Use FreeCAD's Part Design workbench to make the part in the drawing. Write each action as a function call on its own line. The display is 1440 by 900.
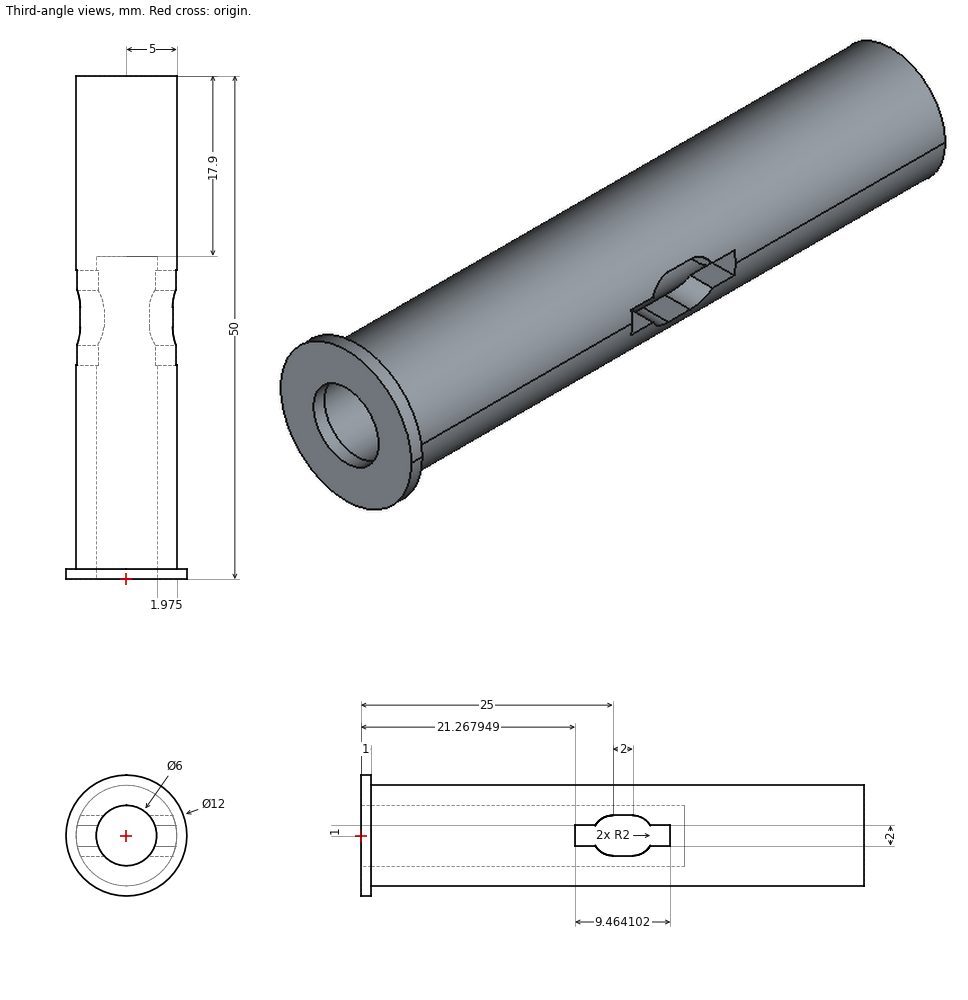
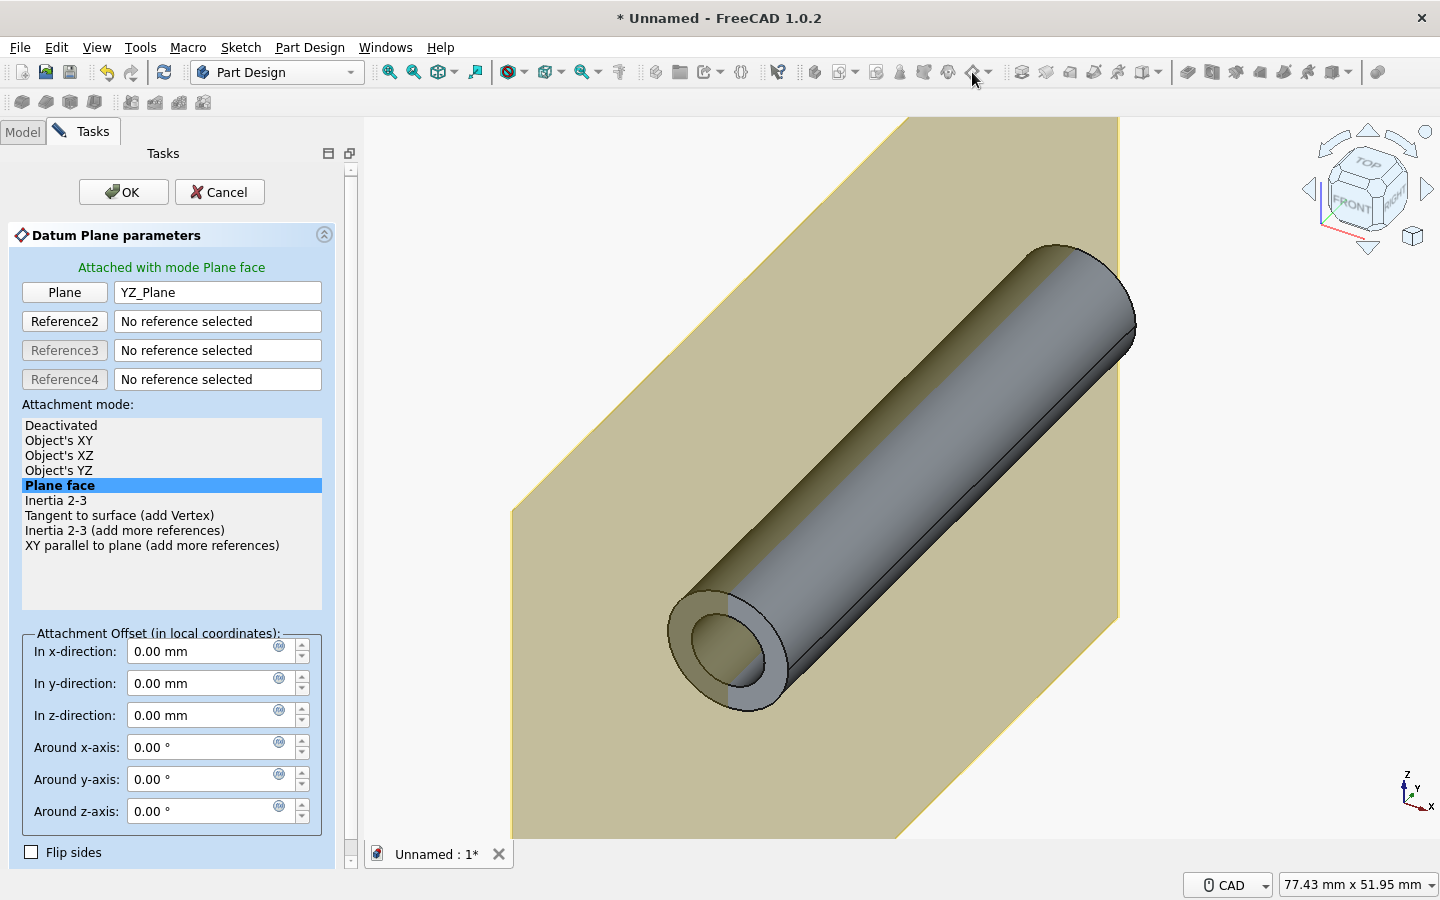
triple_click(210, 715)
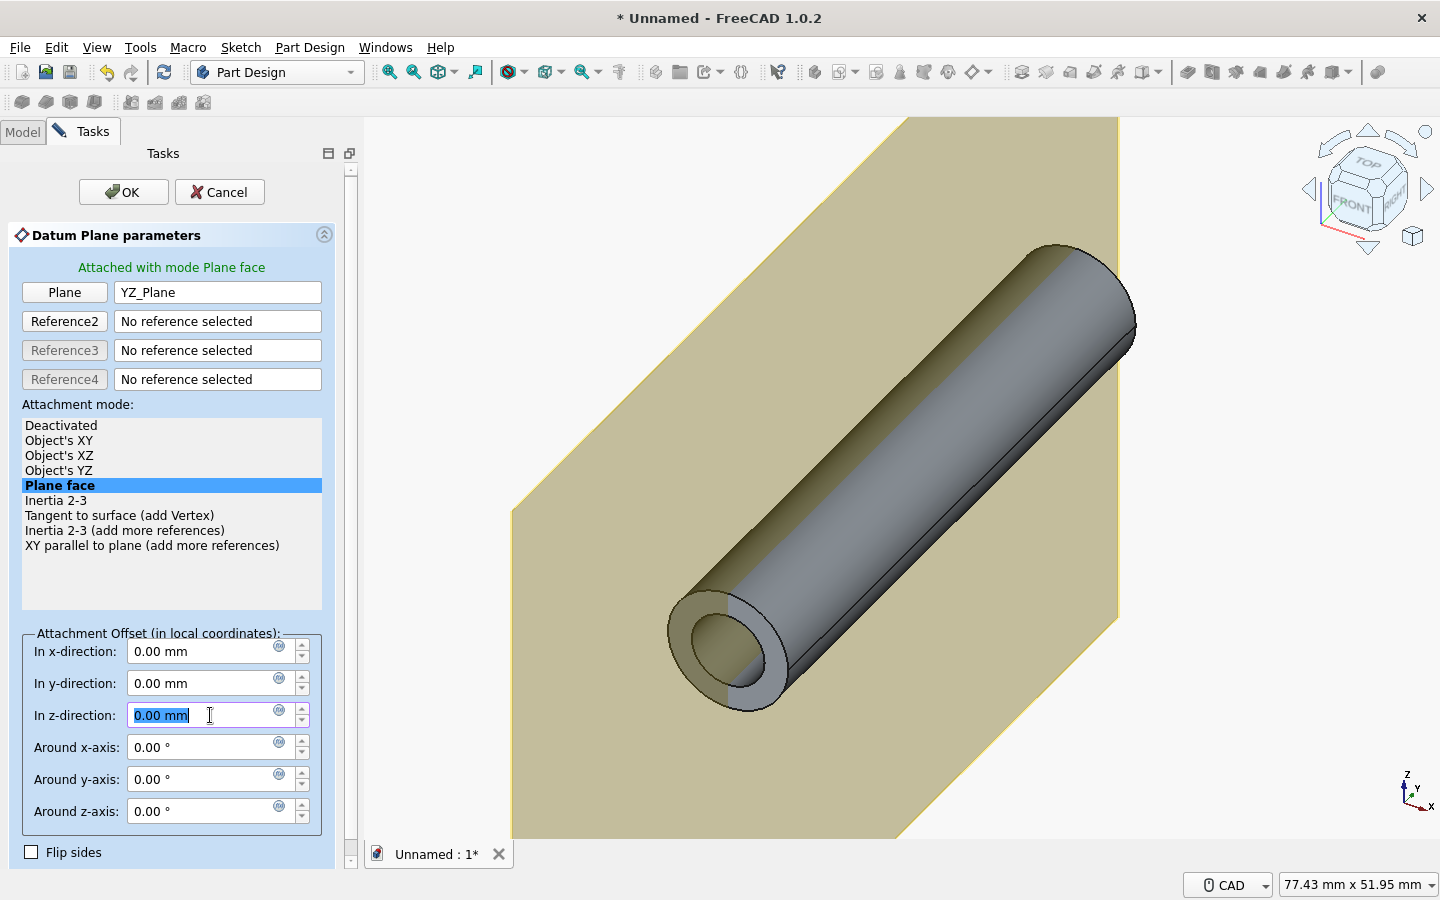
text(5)
key(Tab)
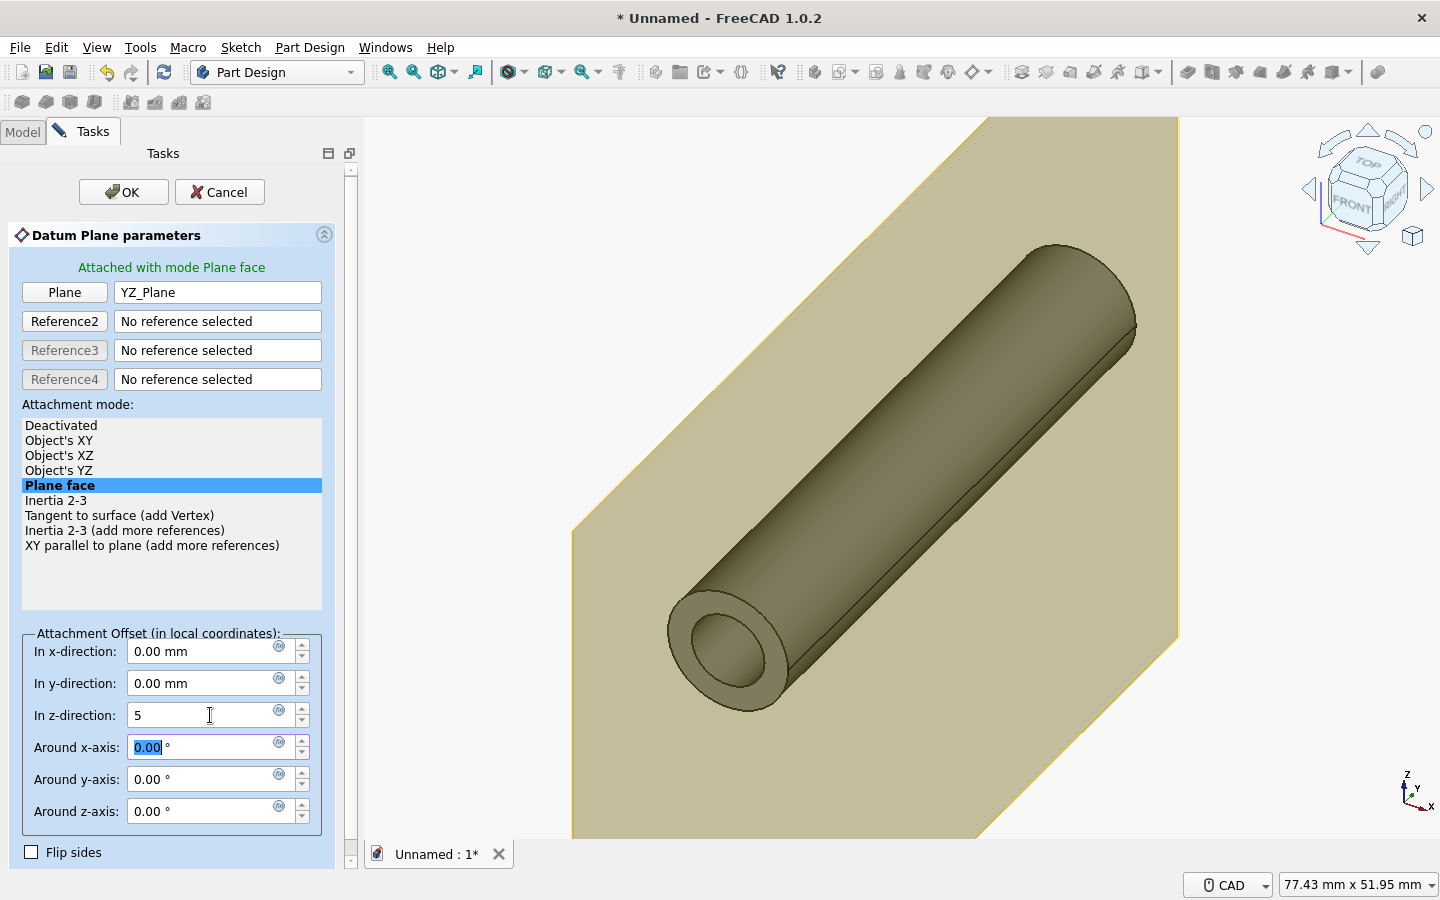
click(124, 192)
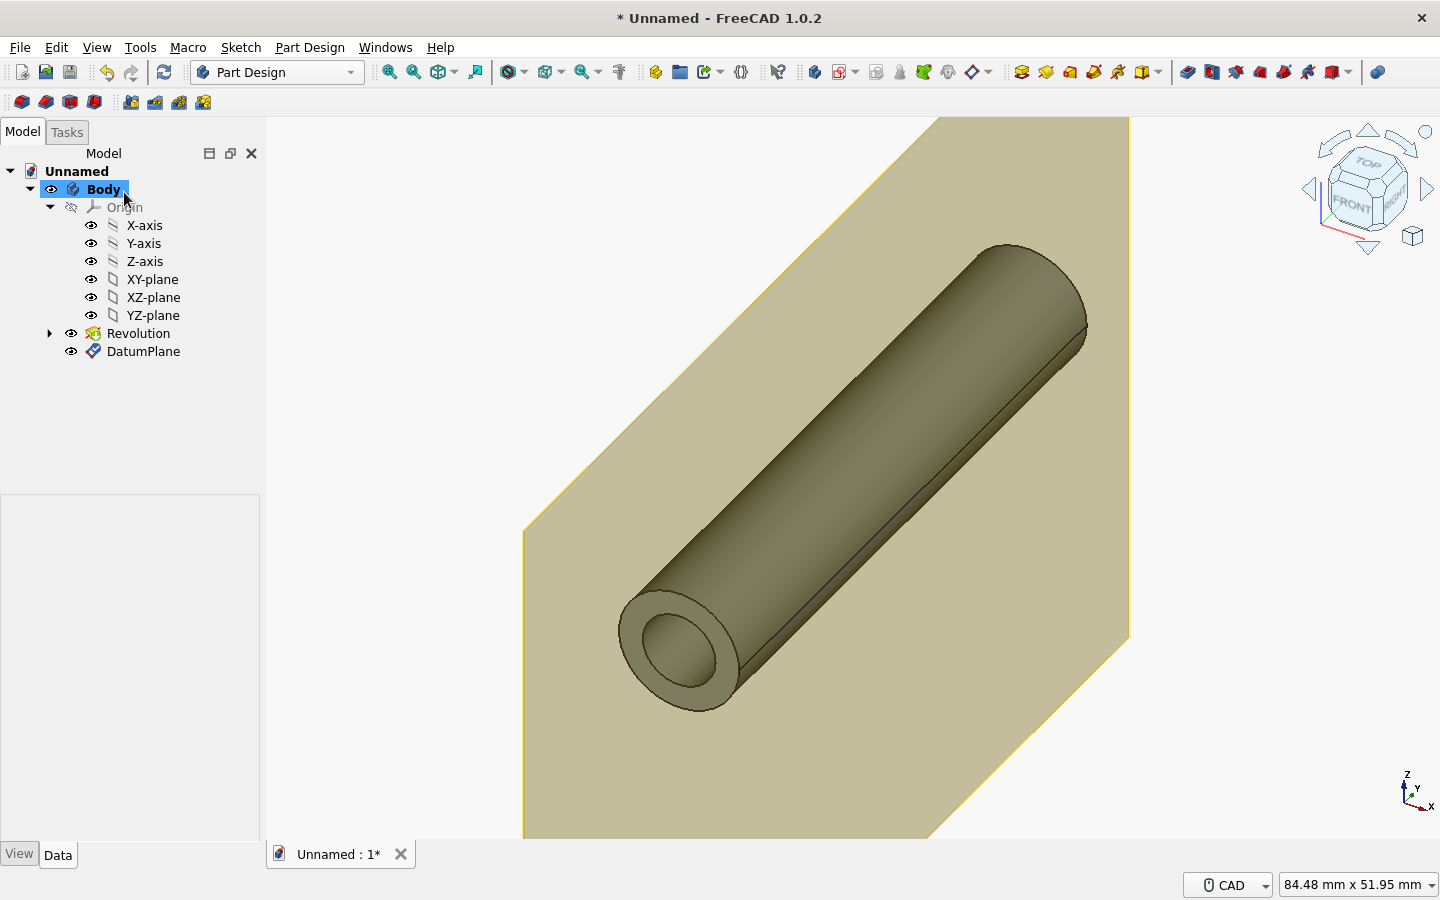
click(116, 351)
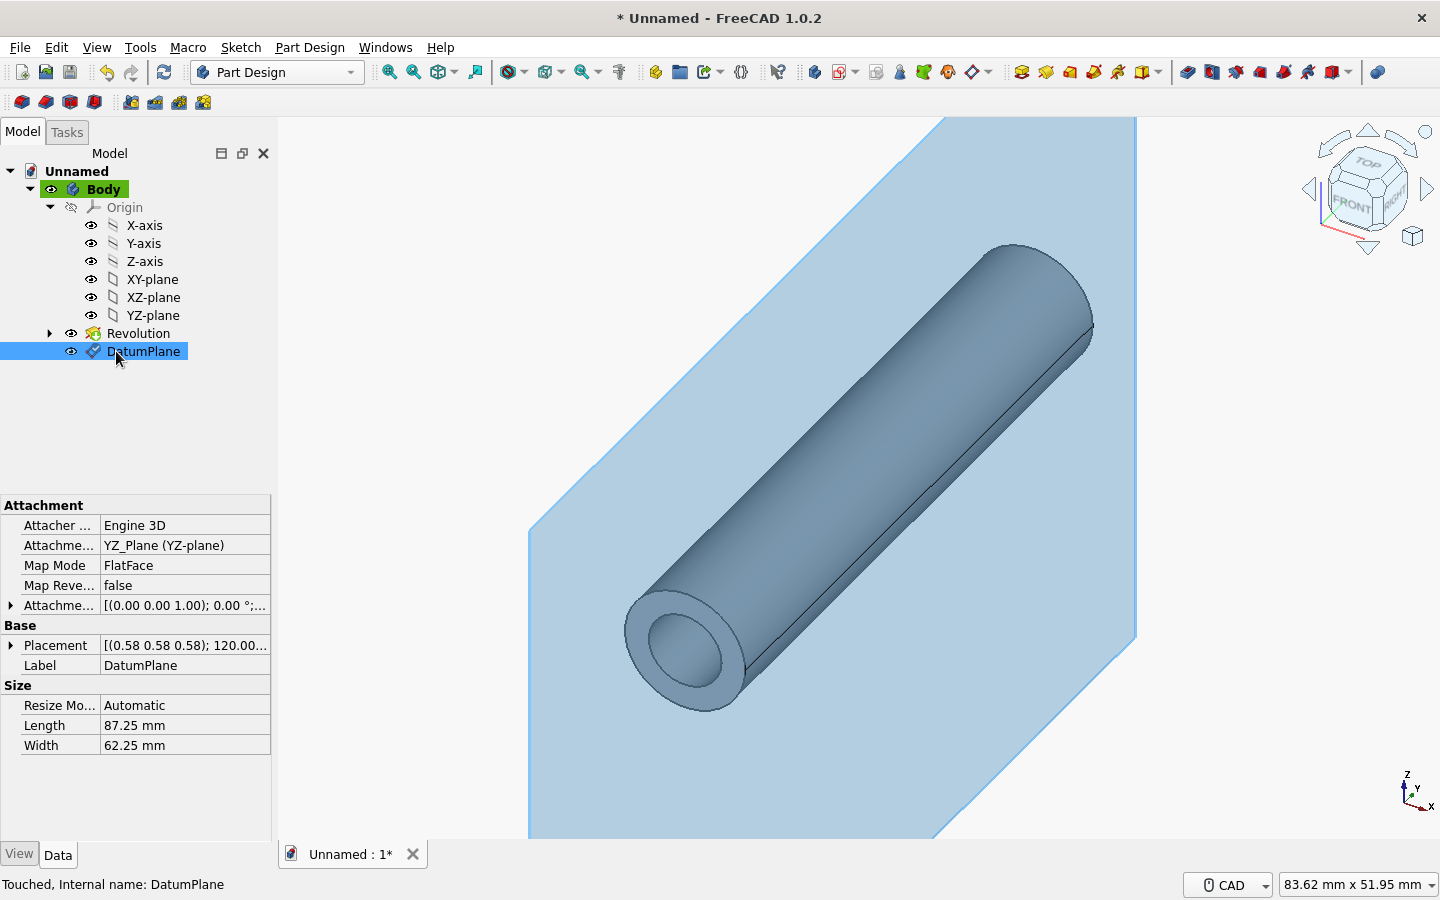
click(840, 72)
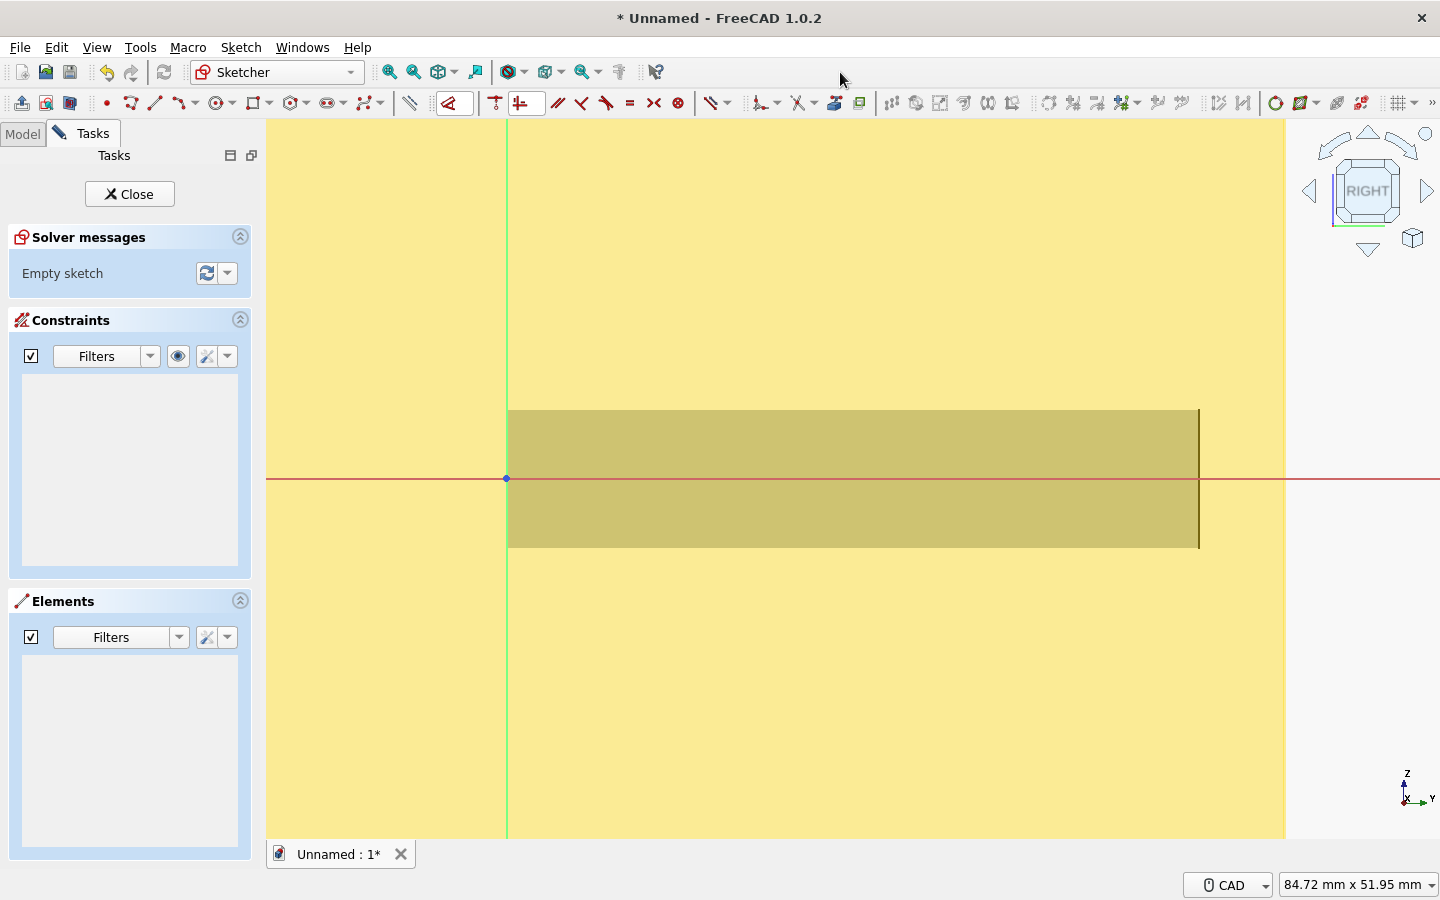
scroll(877, 479, up, 11)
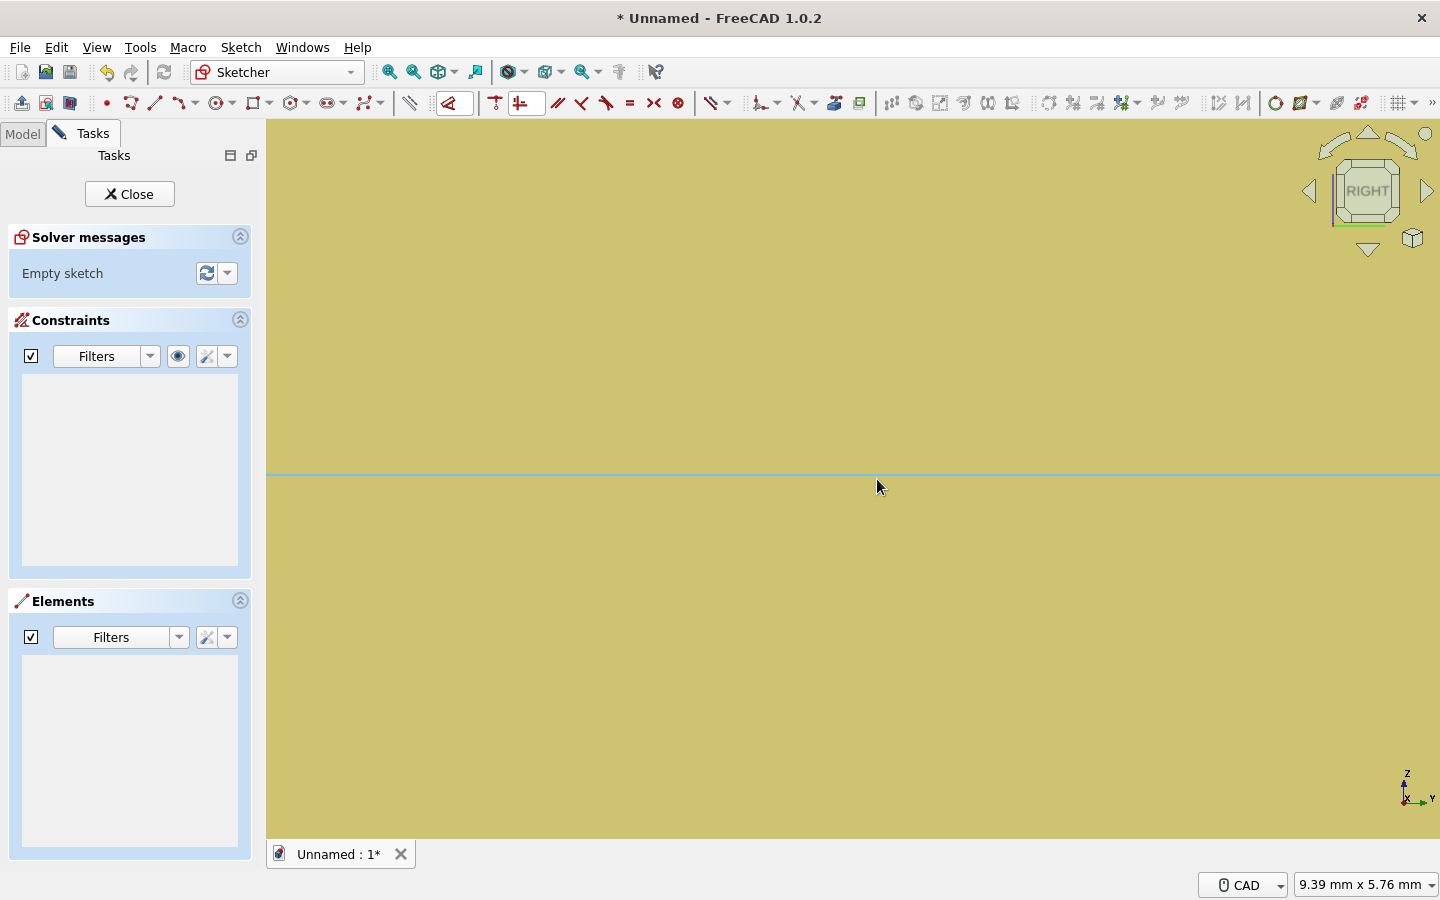
key(g)
key(s)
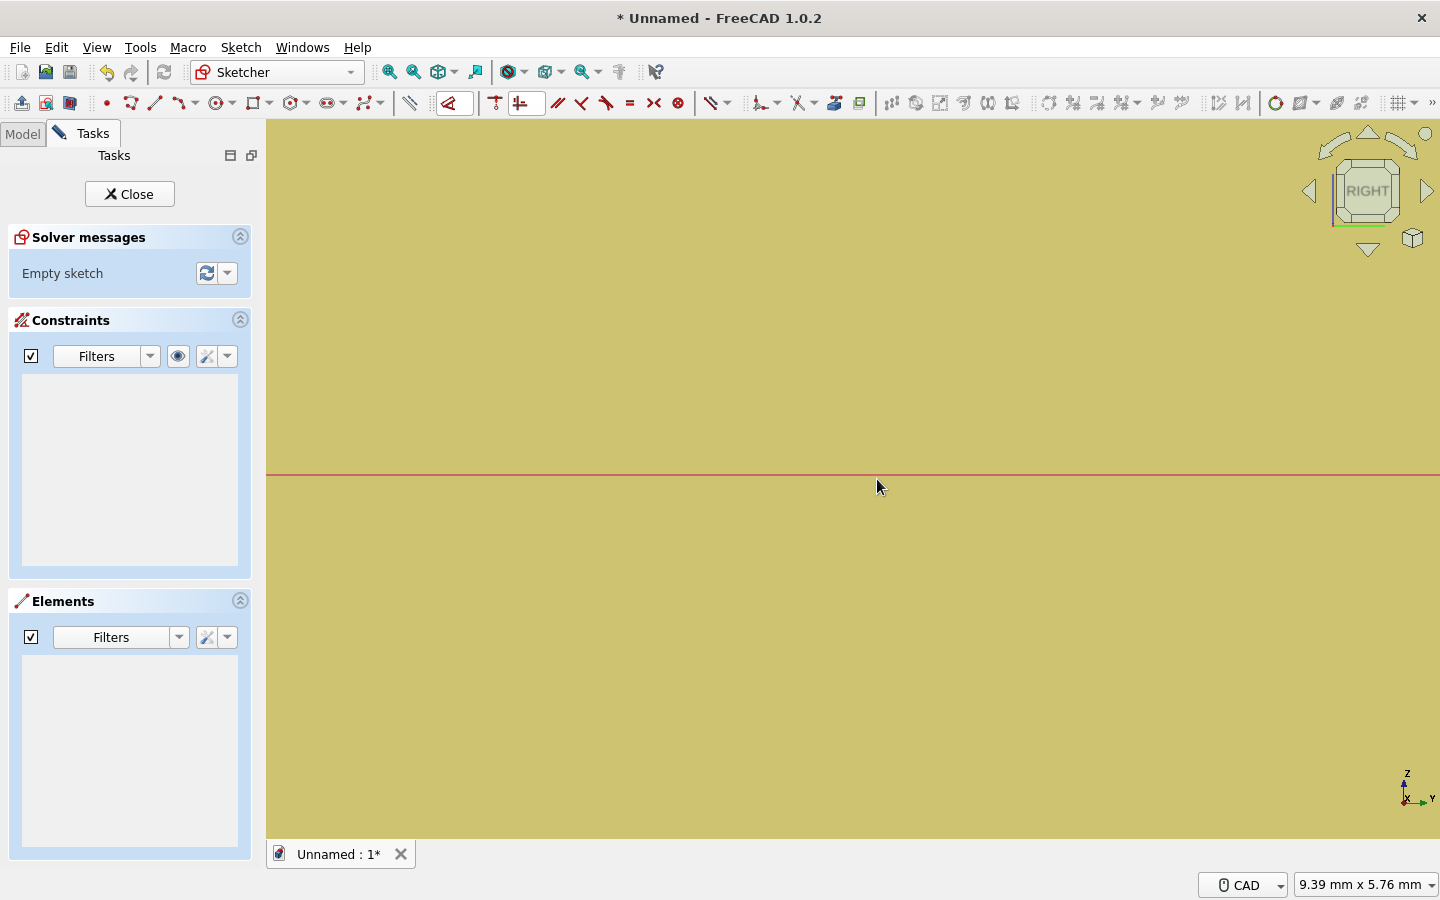
click(656, 475)